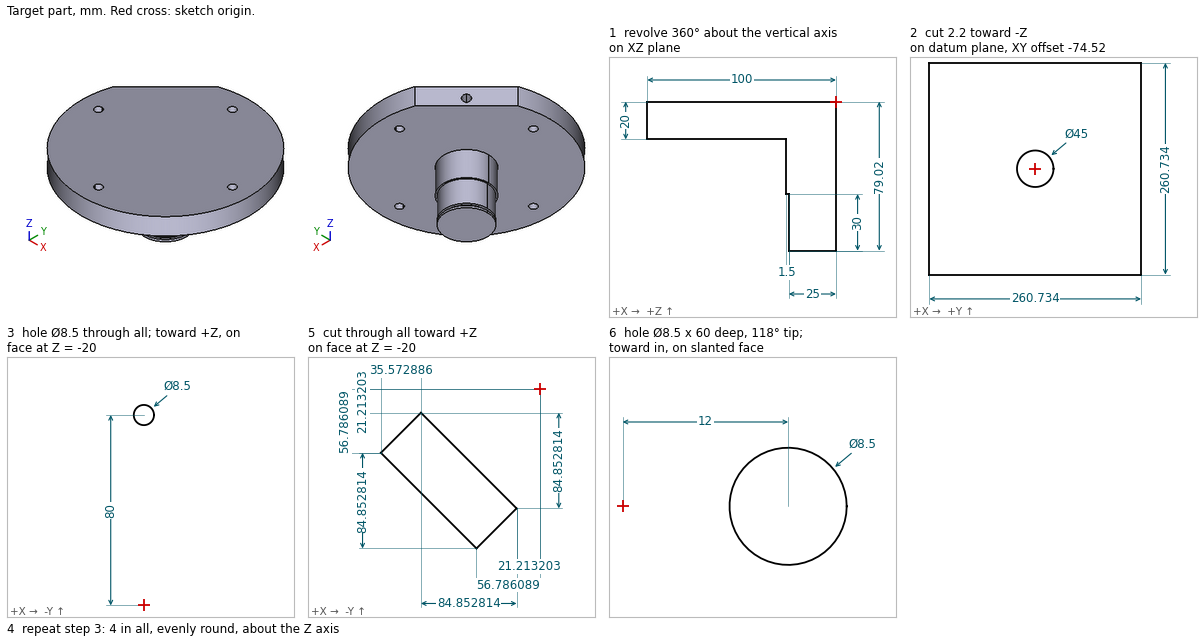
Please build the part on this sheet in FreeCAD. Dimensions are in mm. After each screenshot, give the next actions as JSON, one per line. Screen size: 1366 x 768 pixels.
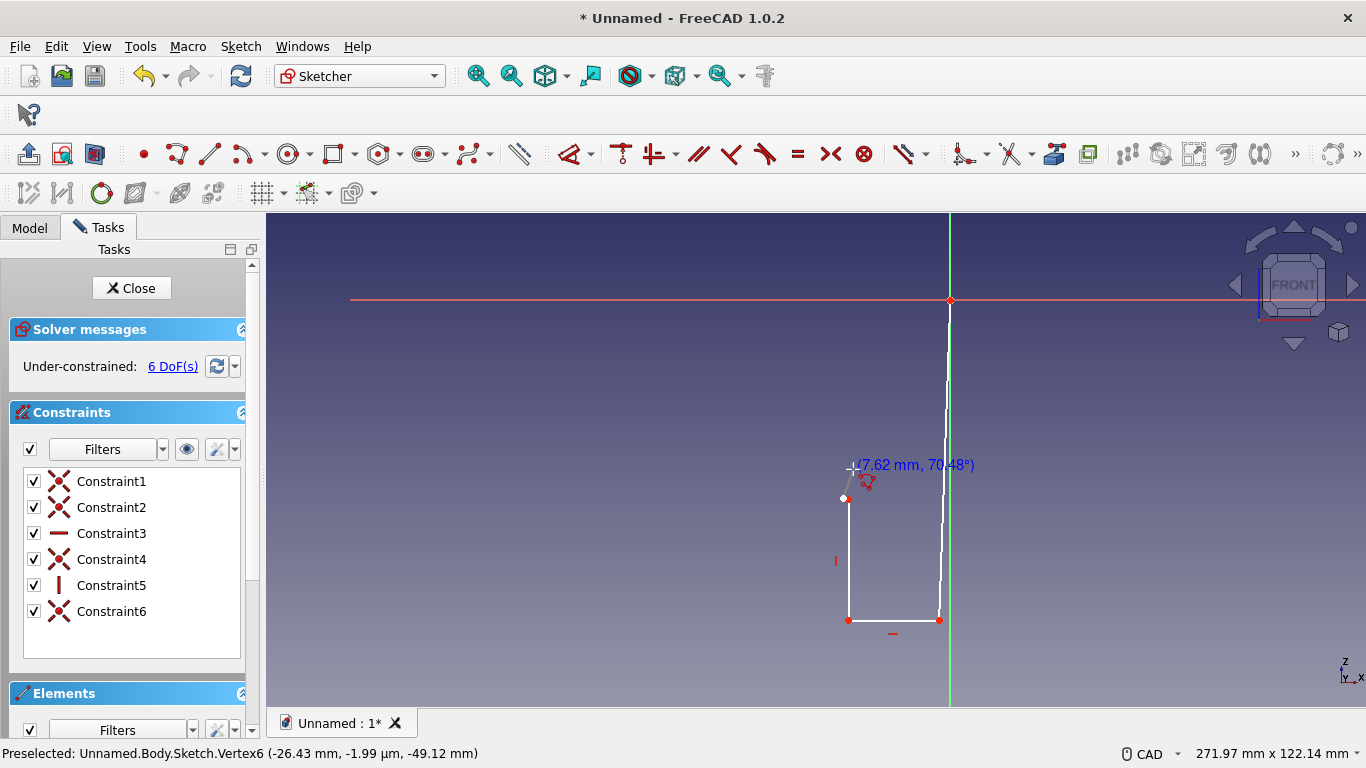
{"action": "left_click", "coordinate": [843, 381]}
{"action": "left_click", "coordinate": [546, 381]}
{"action": "left_click", "coordinate": [546, 309]}
{"action": "left_click", "coordinate": [950, 300]}
{"action": "key", "text": "Escape"}
{"action": "key", "text": "Escape"}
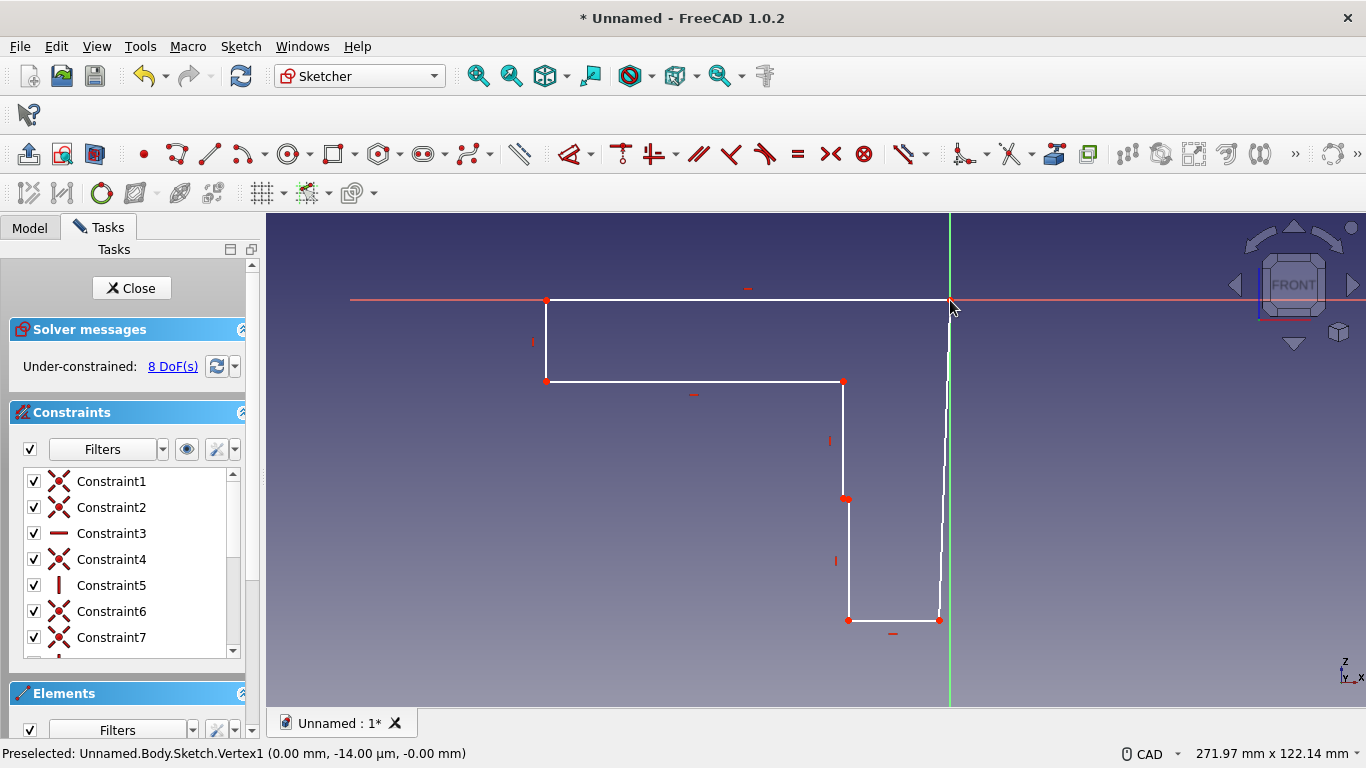
{"action": "left_click", "coordinate": [947, 397]}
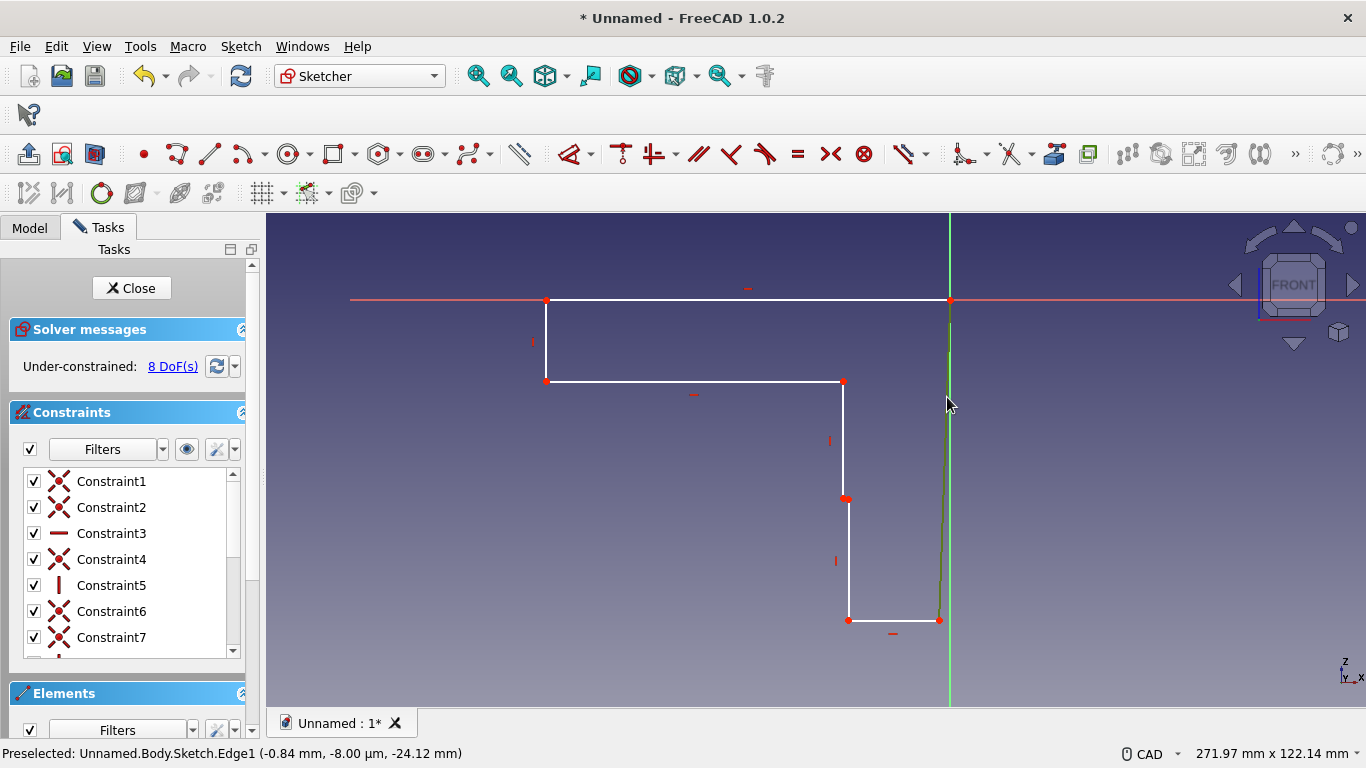
{"action": "key", "text": "v"}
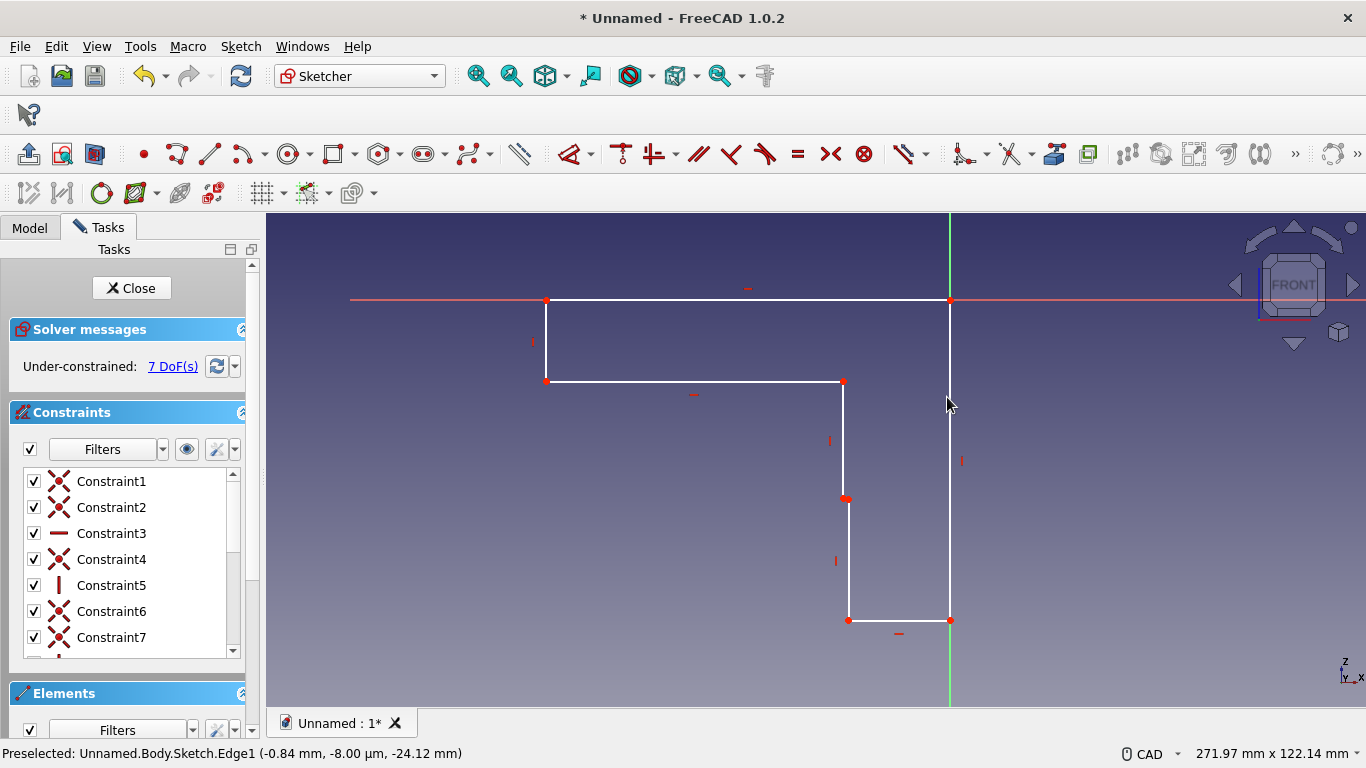
{"action": "scroll", "coordinate": [846, 499], "scroll_direction": "up", "scroll_amount": 8}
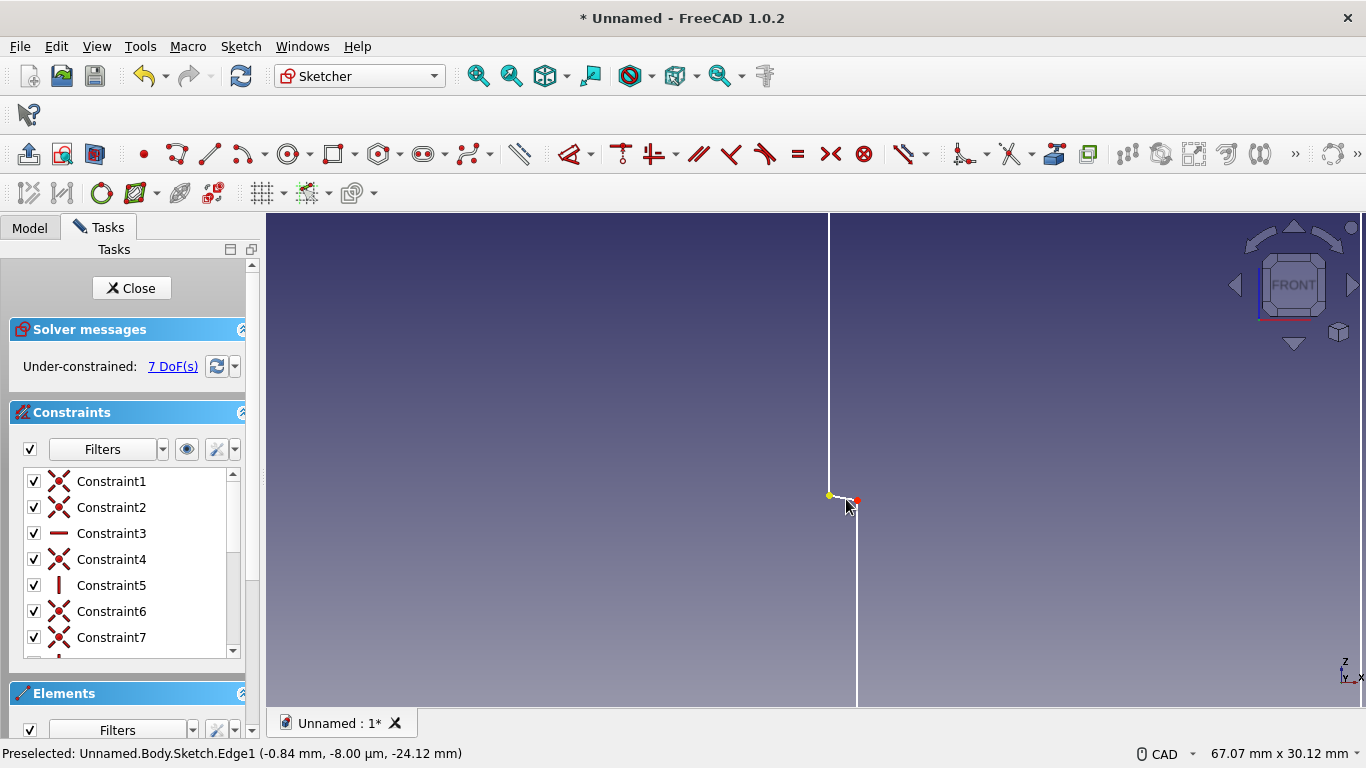
{"action": "left_click", "coordinate": [843, 498]}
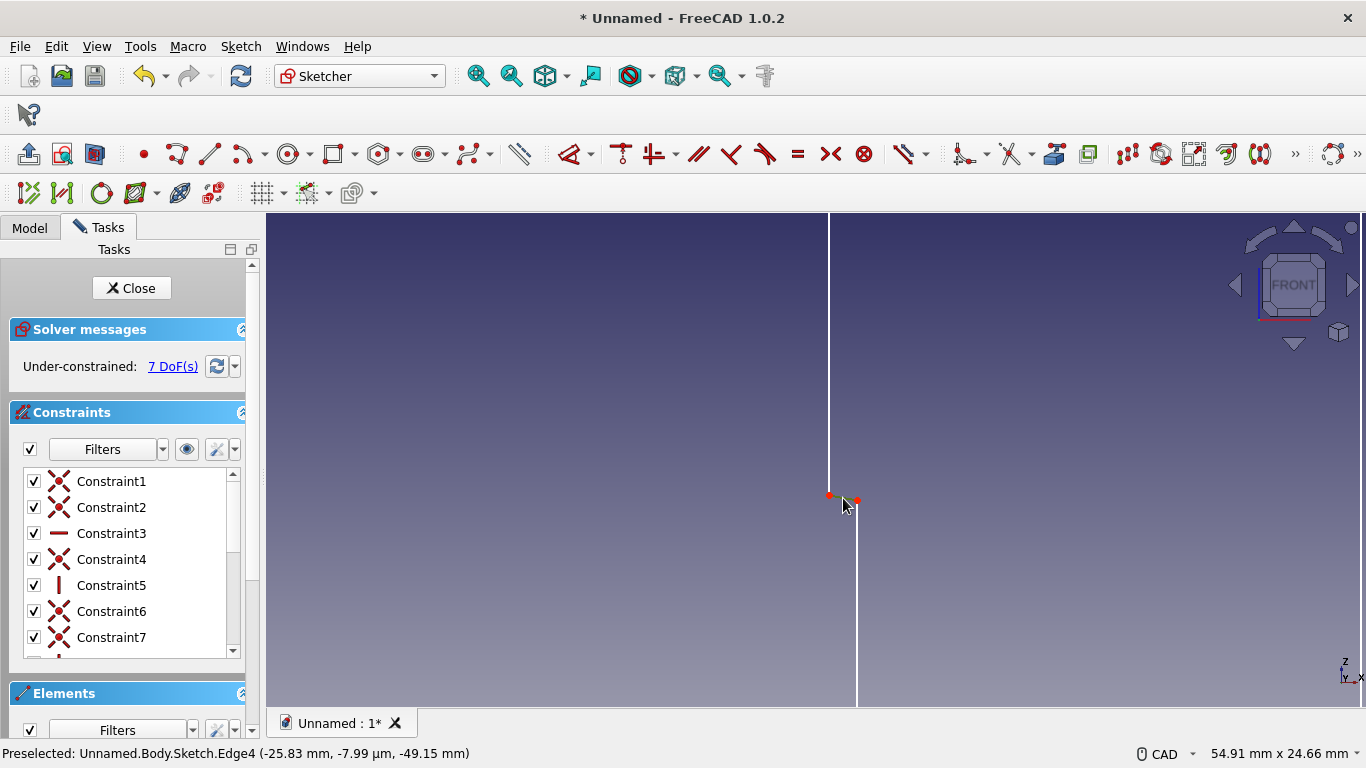
{"action": "left_click", "coordinate": [676, 154]}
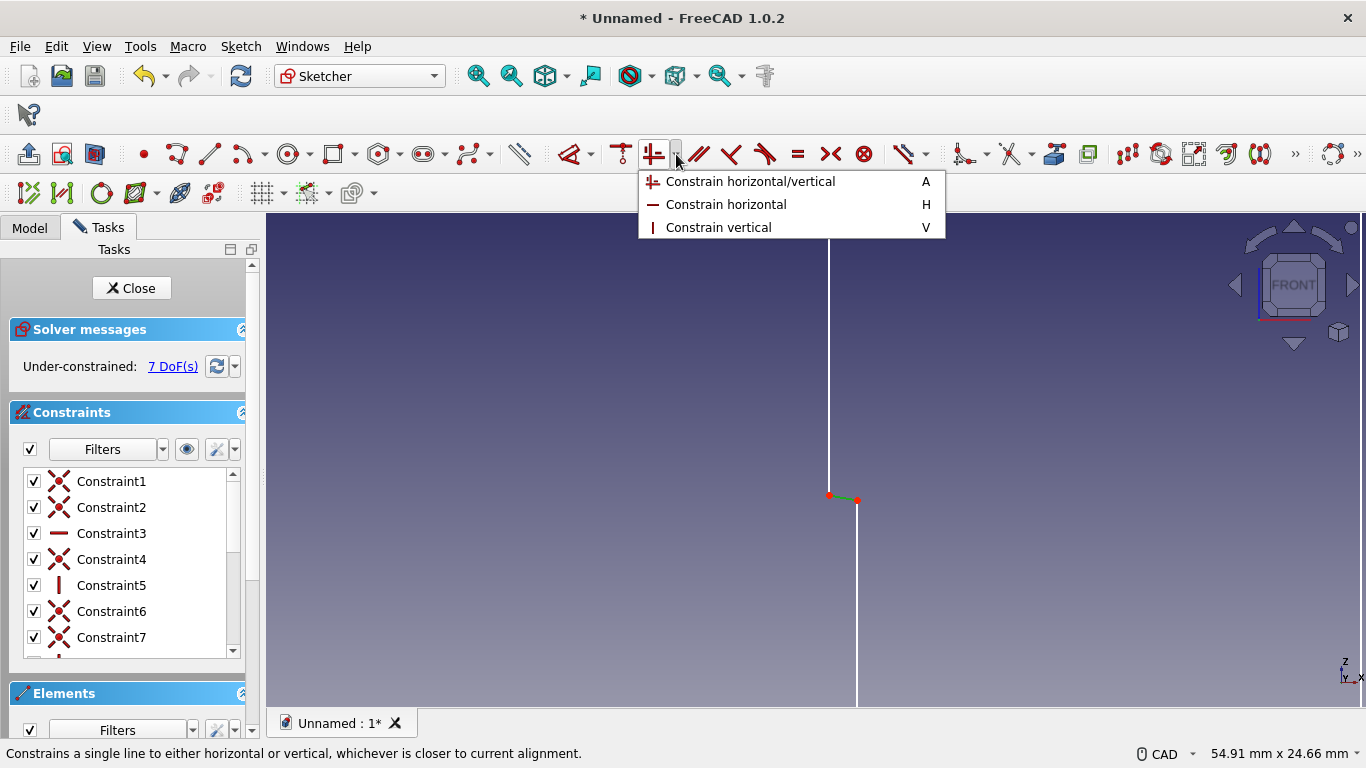
{"action": "left_click", "coordinate": [792, 204]}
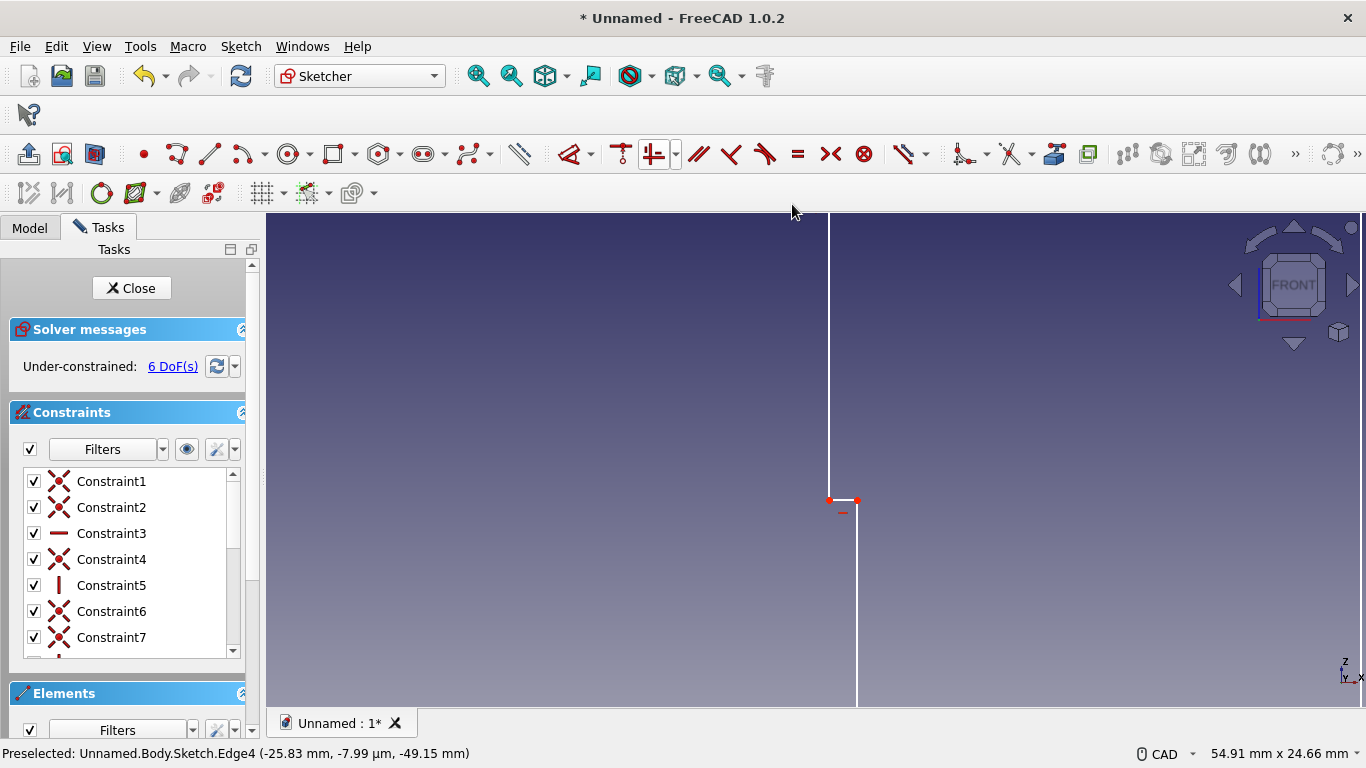
{"action": "left_click", "coordinate": [568, 154]}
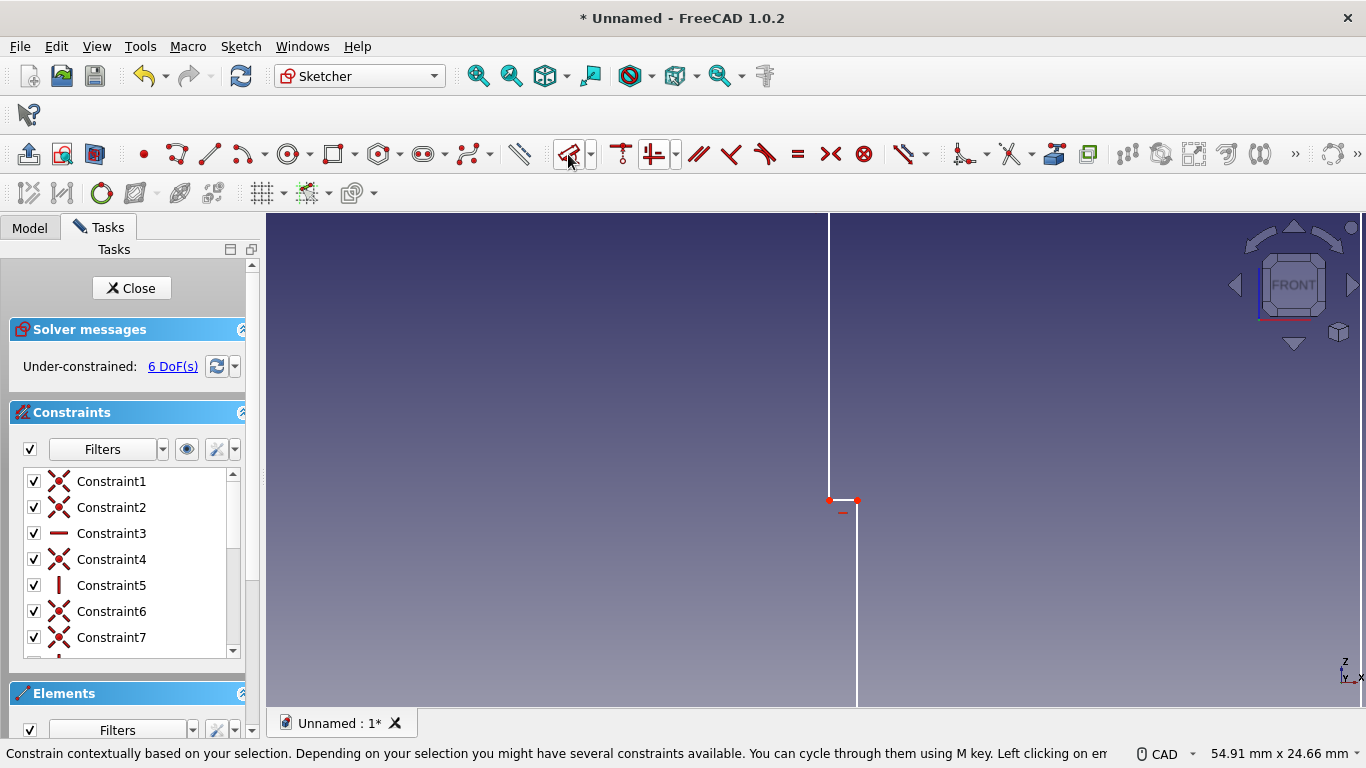
{"action": "scroll", "coordinate": [846, 499], "scroll_direction": "down", "scroll_amount": 8}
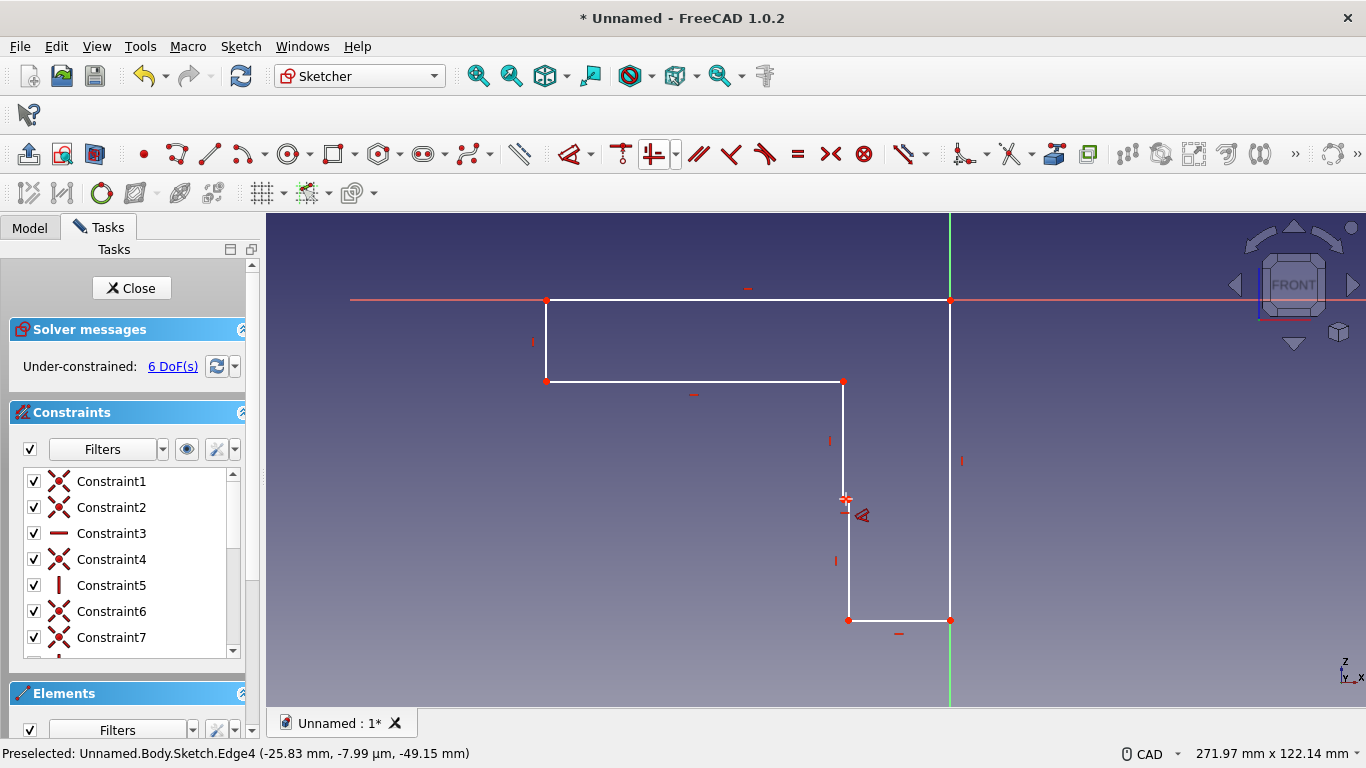
{"action": "left_click", "coordinate": [920, 621]}
{"action": "left_click", "coordinate": [900, 655]}